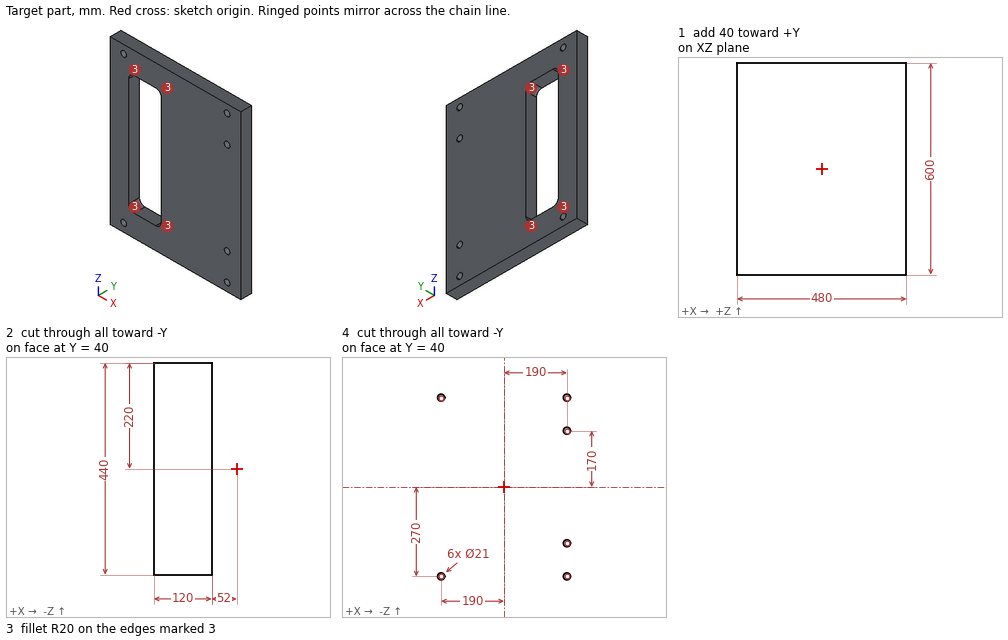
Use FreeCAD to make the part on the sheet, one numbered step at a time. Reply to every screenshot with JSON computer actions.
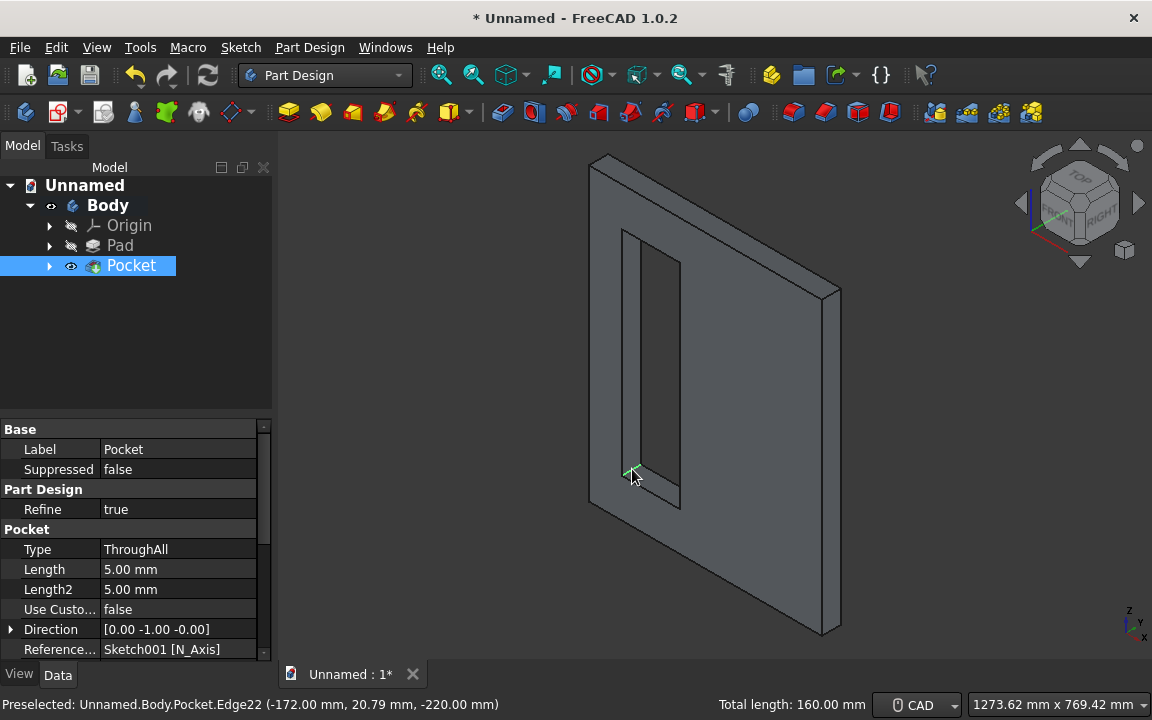
{"action": "left_click", "coordinate": [794, 112]}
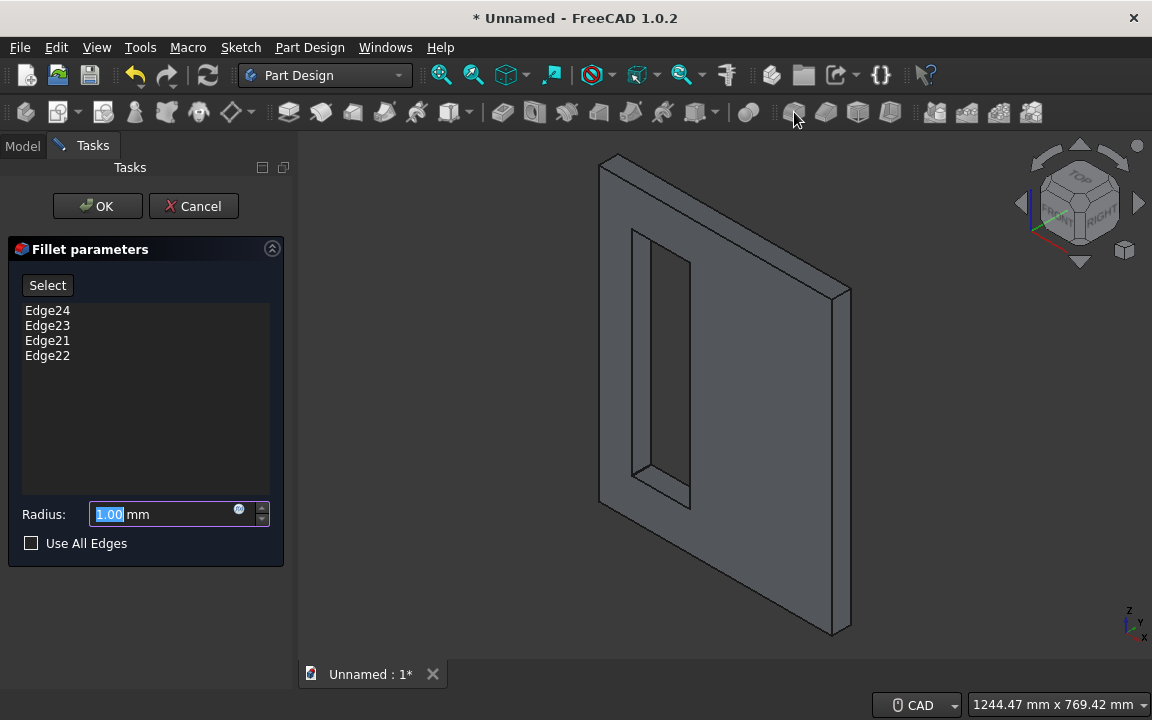
{"action": "type", "text": "20"}
{"action": "key", "text": "Tab"}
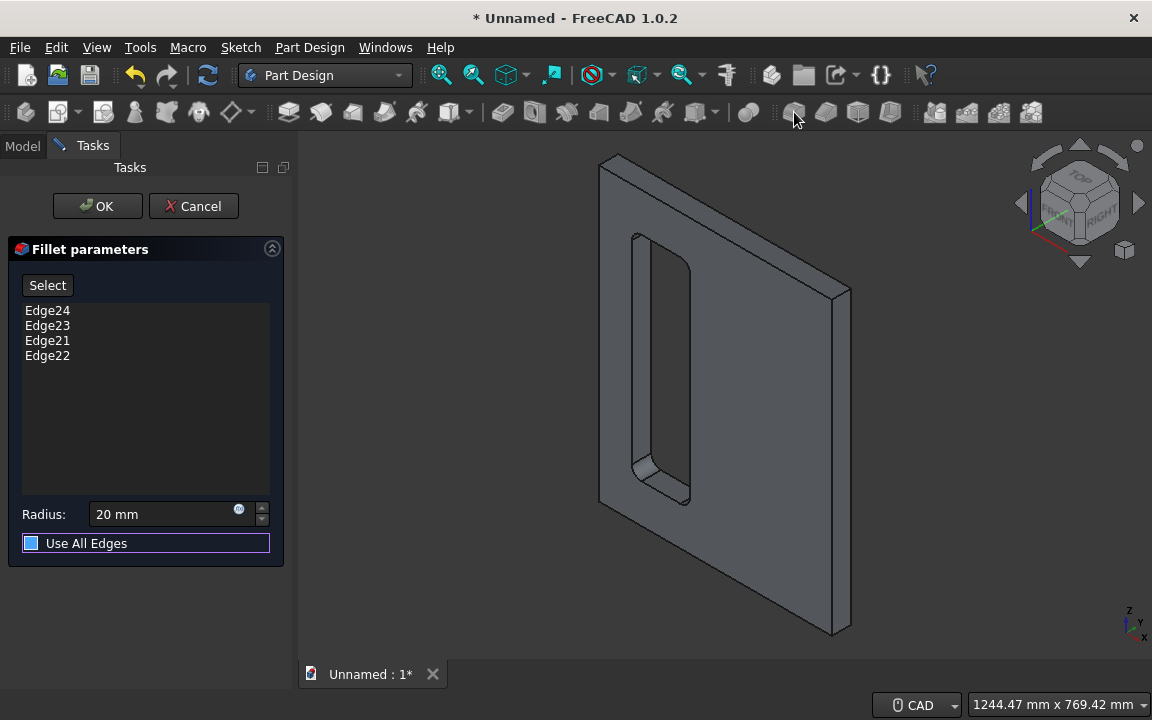
{"action": "left_click", "coordinate": [98, 206]}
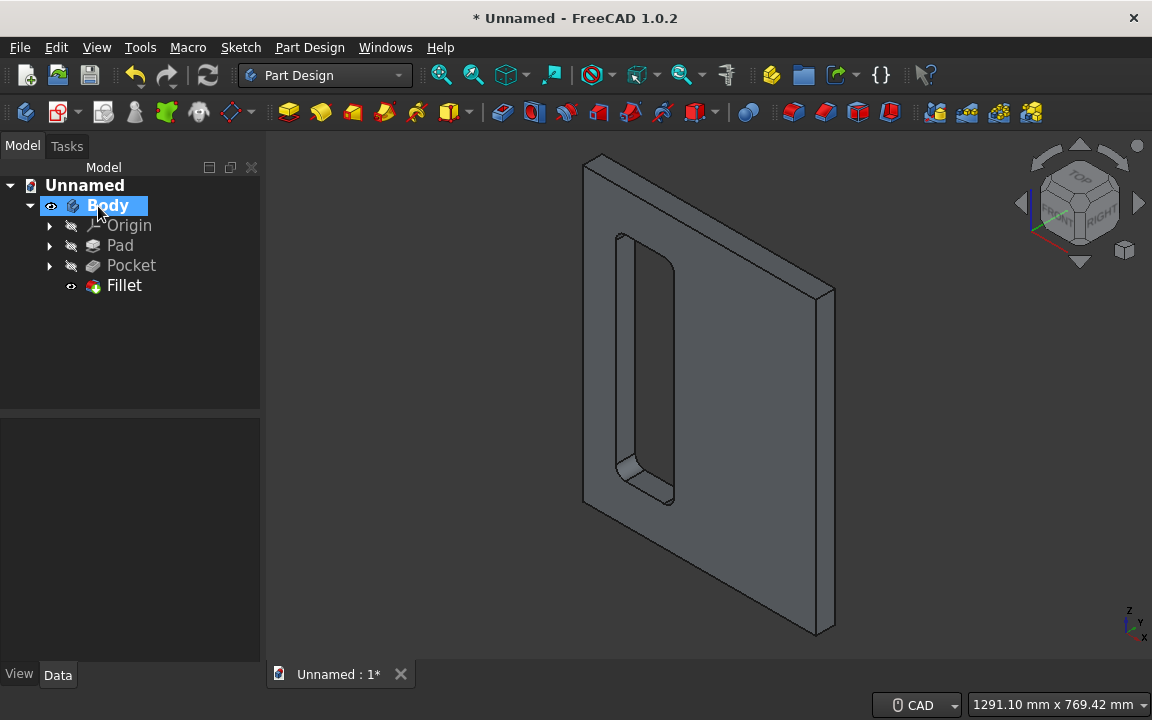
{"action": "key", "text": "4"}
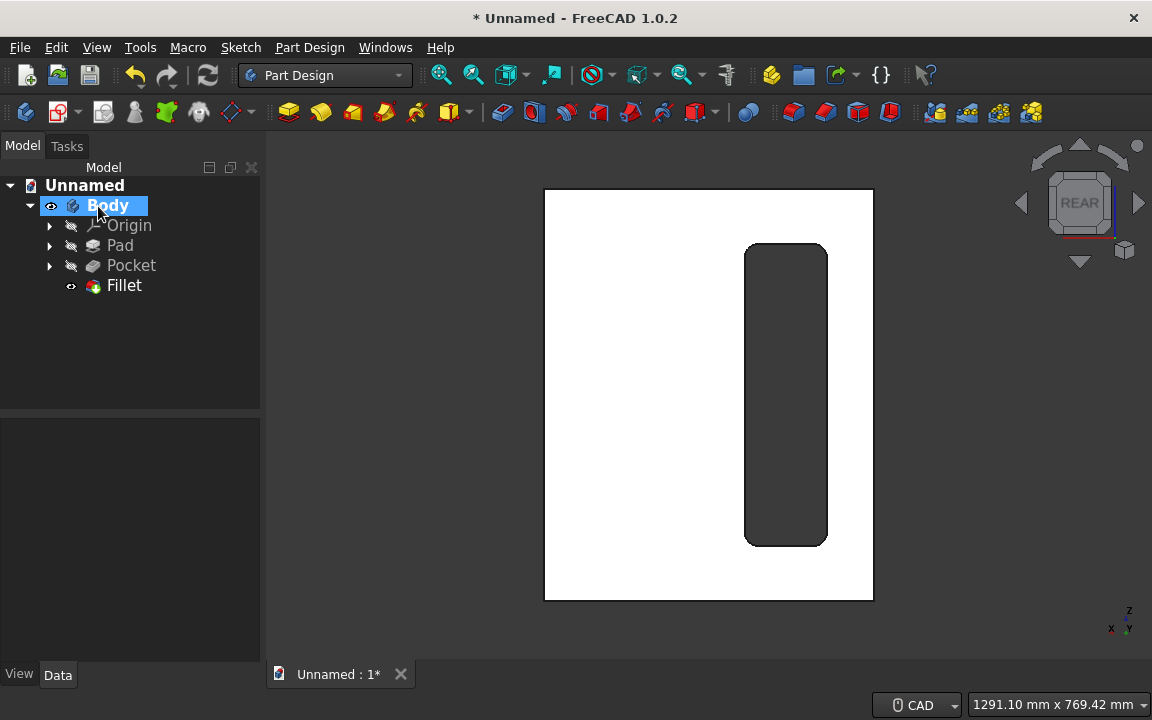
{"action": "left_click", "coordinate": [662, 276]}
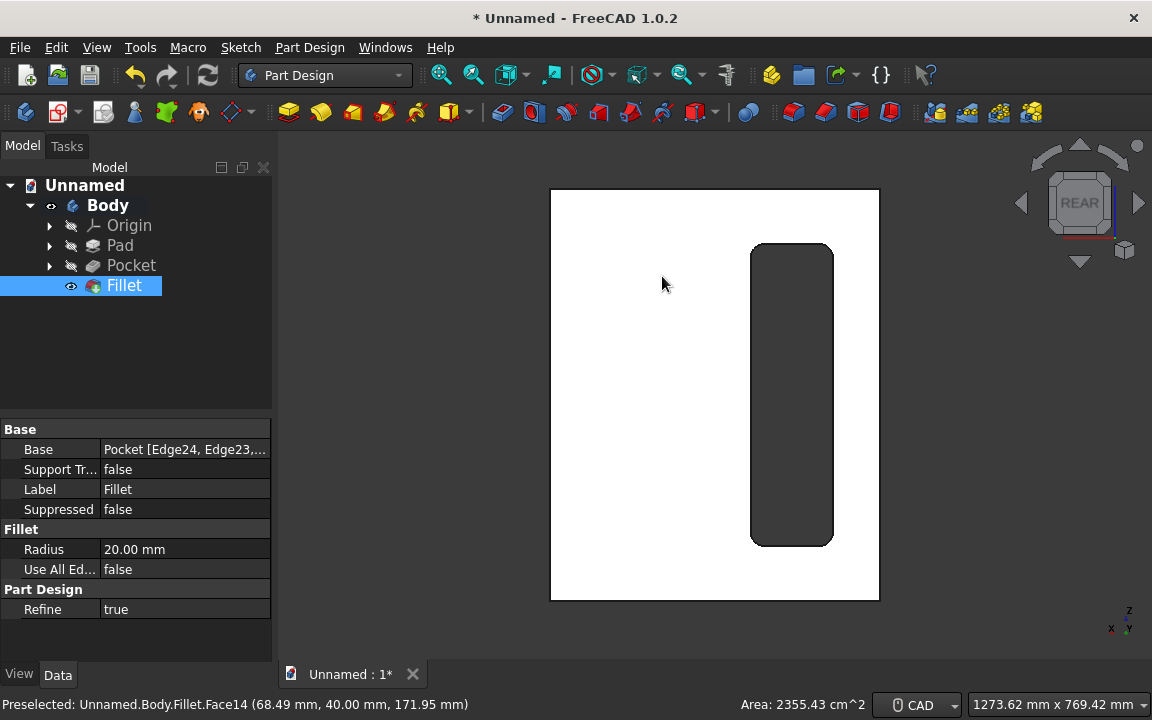
{"action": "left_click", "coordinate": [58, 112]}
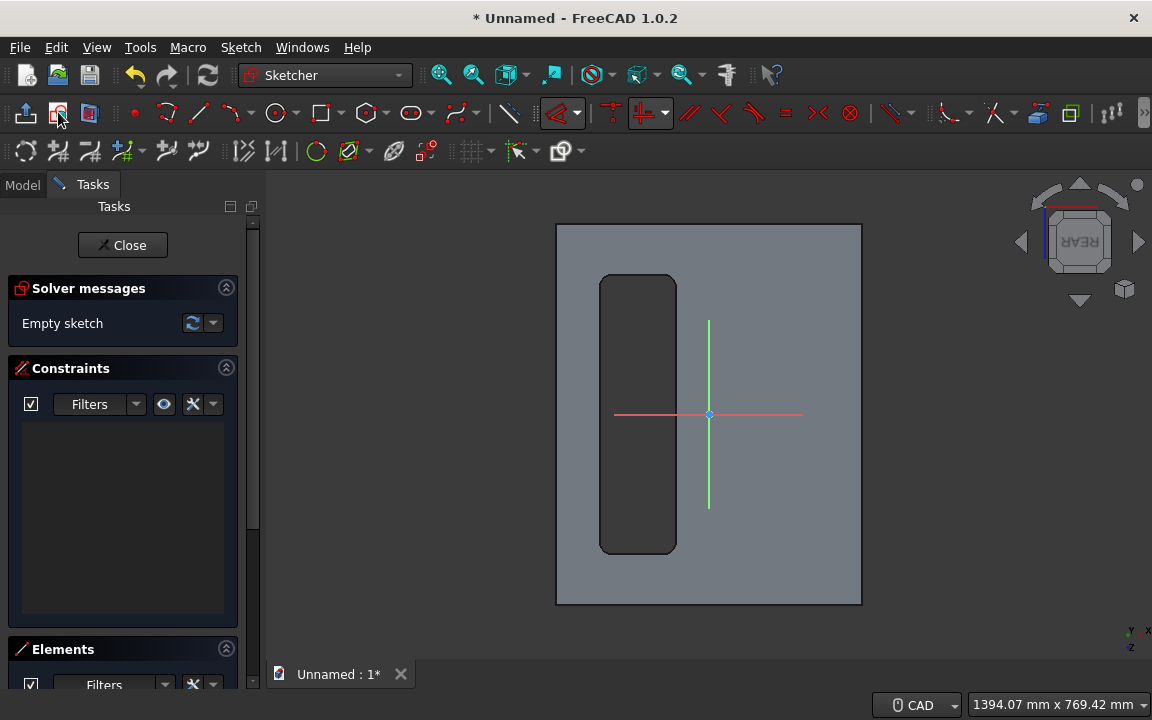
{"action": "left_click", "coordinate": [276, 114]}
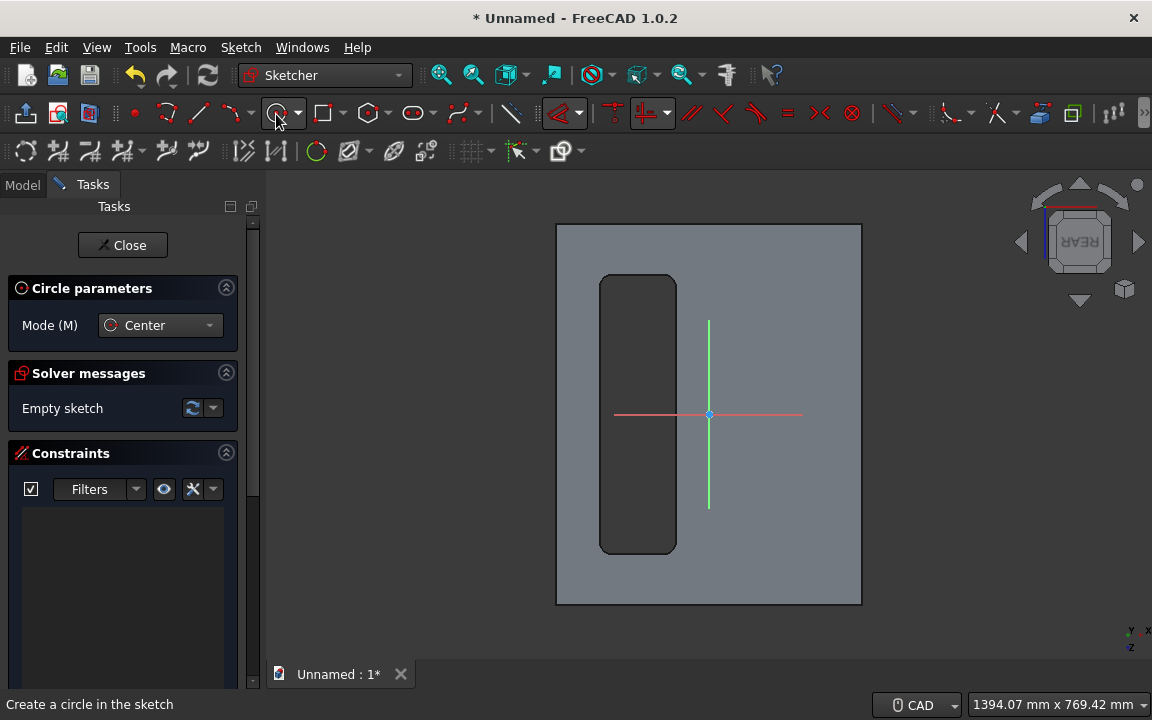
{"action": "scroll", "coordinate": [588, 586], "scroll_direction": "up", "scroll_amount": 7}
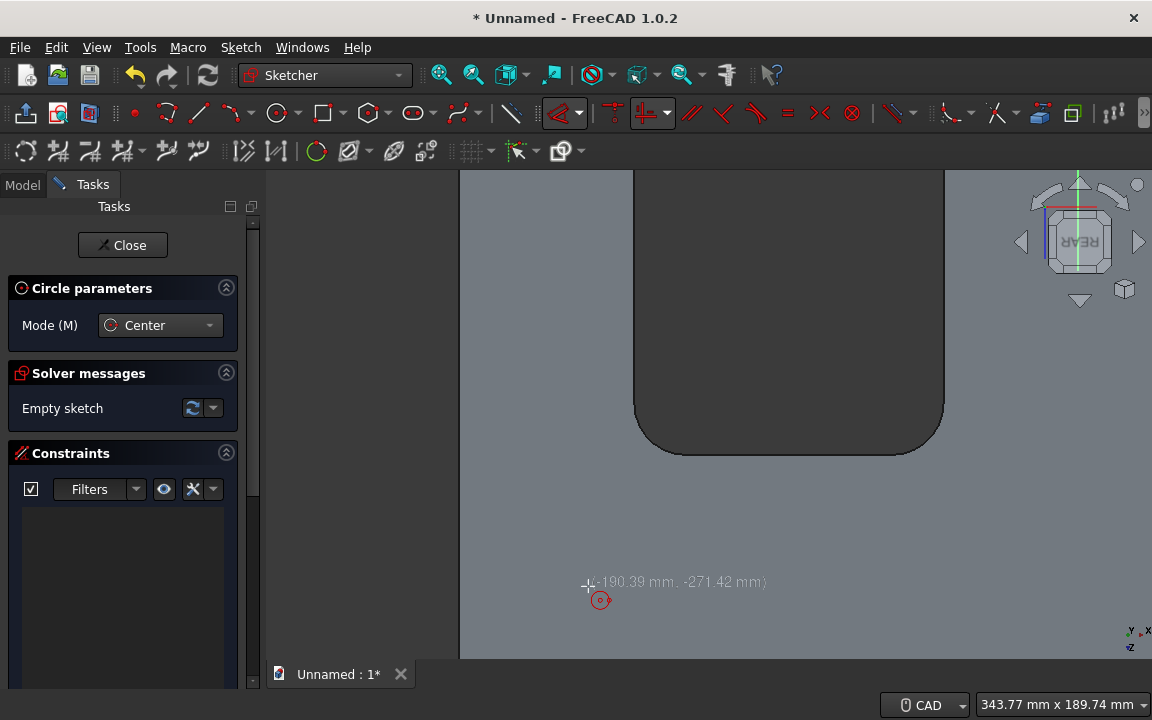
{"action": "scroll", "coordinate": [530, 548], "scroll_direction": "down", "scroll_amount": 8}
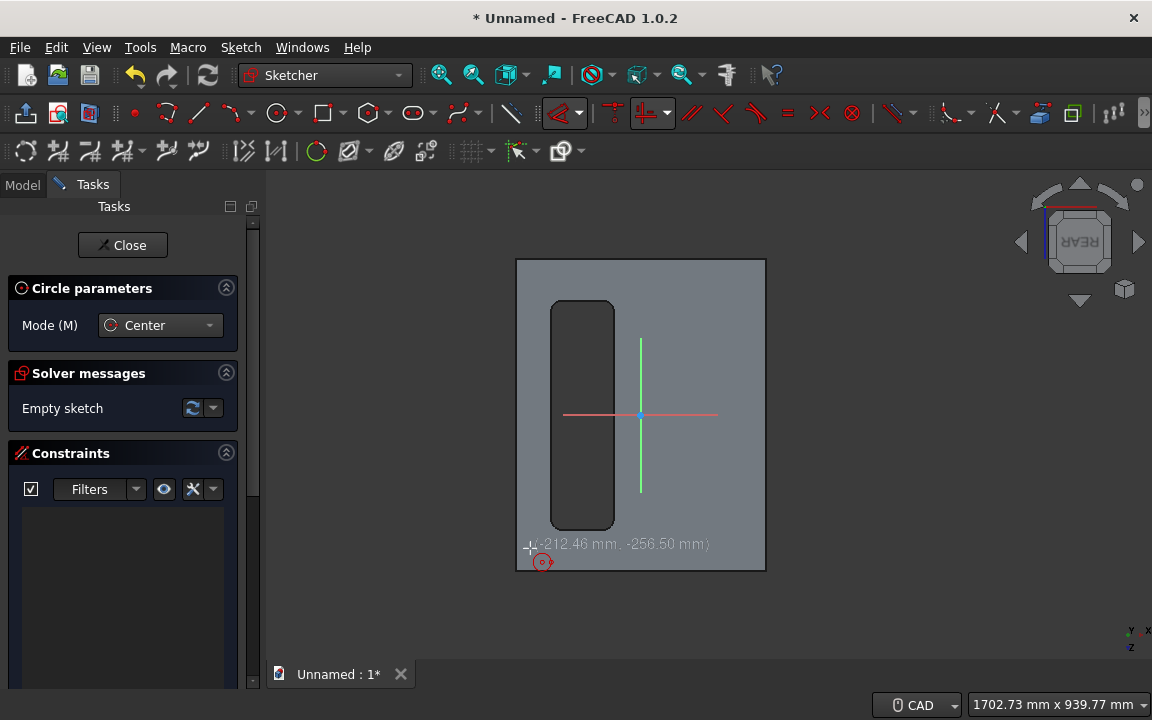
{"action": "left_click", "coordinate": [542, 556]}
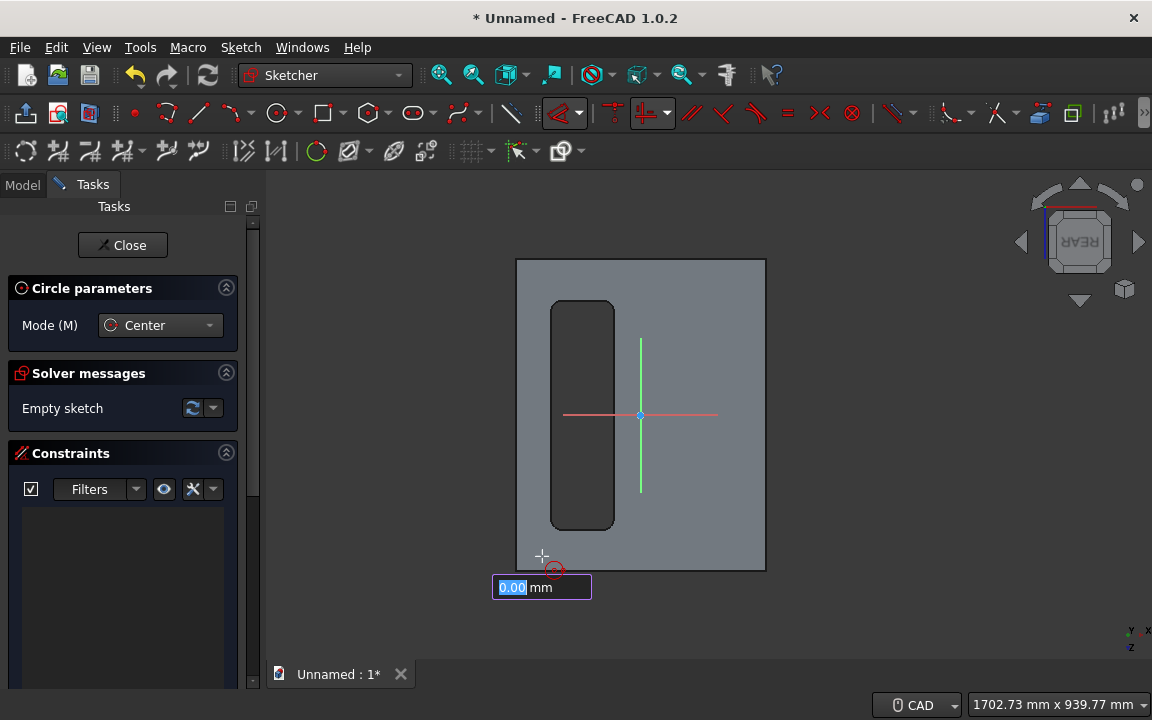
{"action": "scroll", "coordinate": [546, 552], "scroll_direction": "up", "scroll_amount": 6}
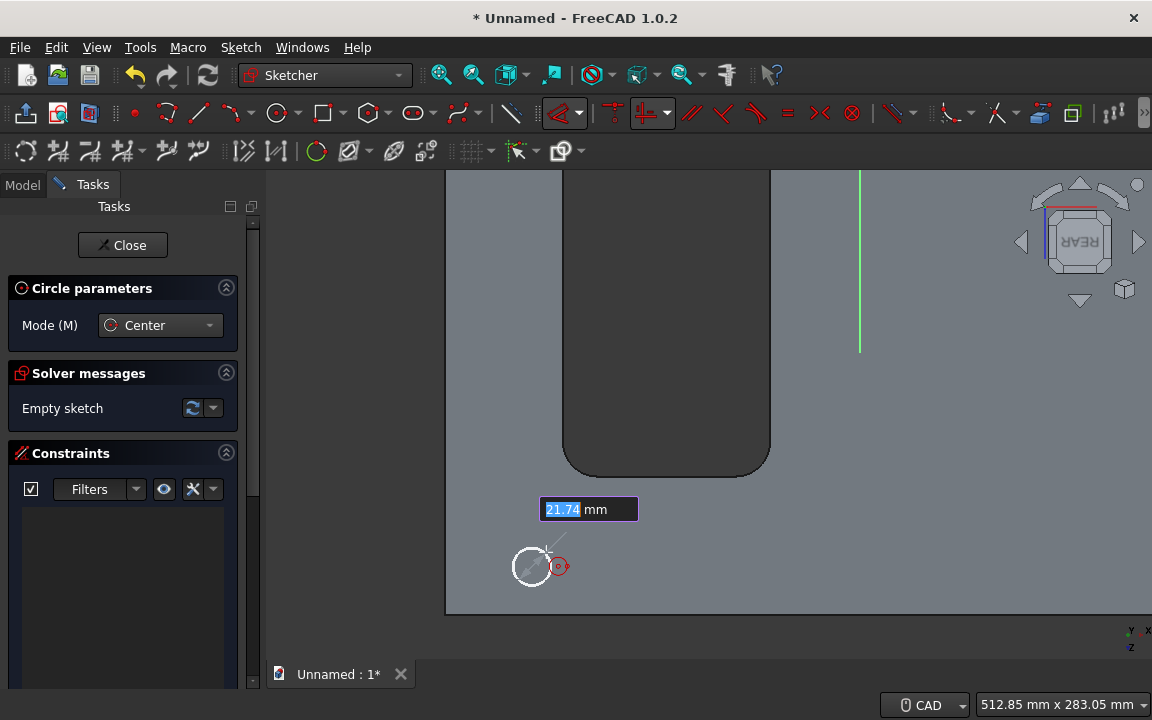
{"action": "left_click", "coordinate": [545, 550]}